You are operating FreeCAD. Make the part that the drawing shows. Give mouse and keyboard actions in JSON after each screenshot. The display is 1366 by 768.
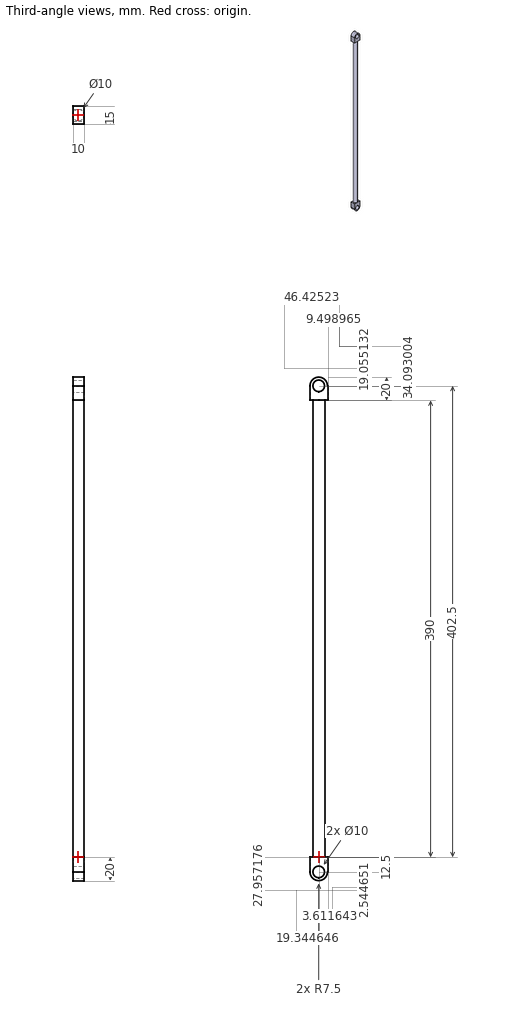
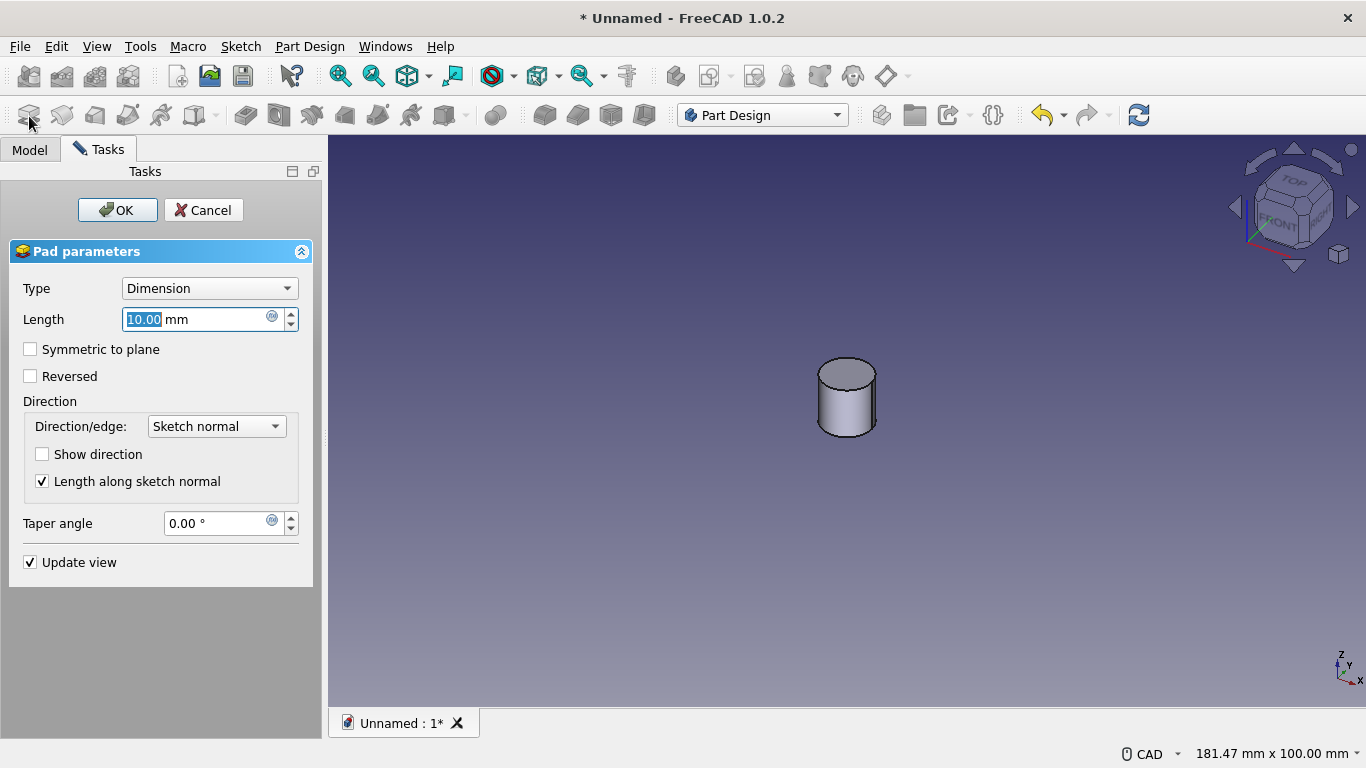
{"action": "type", "text": "390"}
{"action": "key", "text": "Tab"}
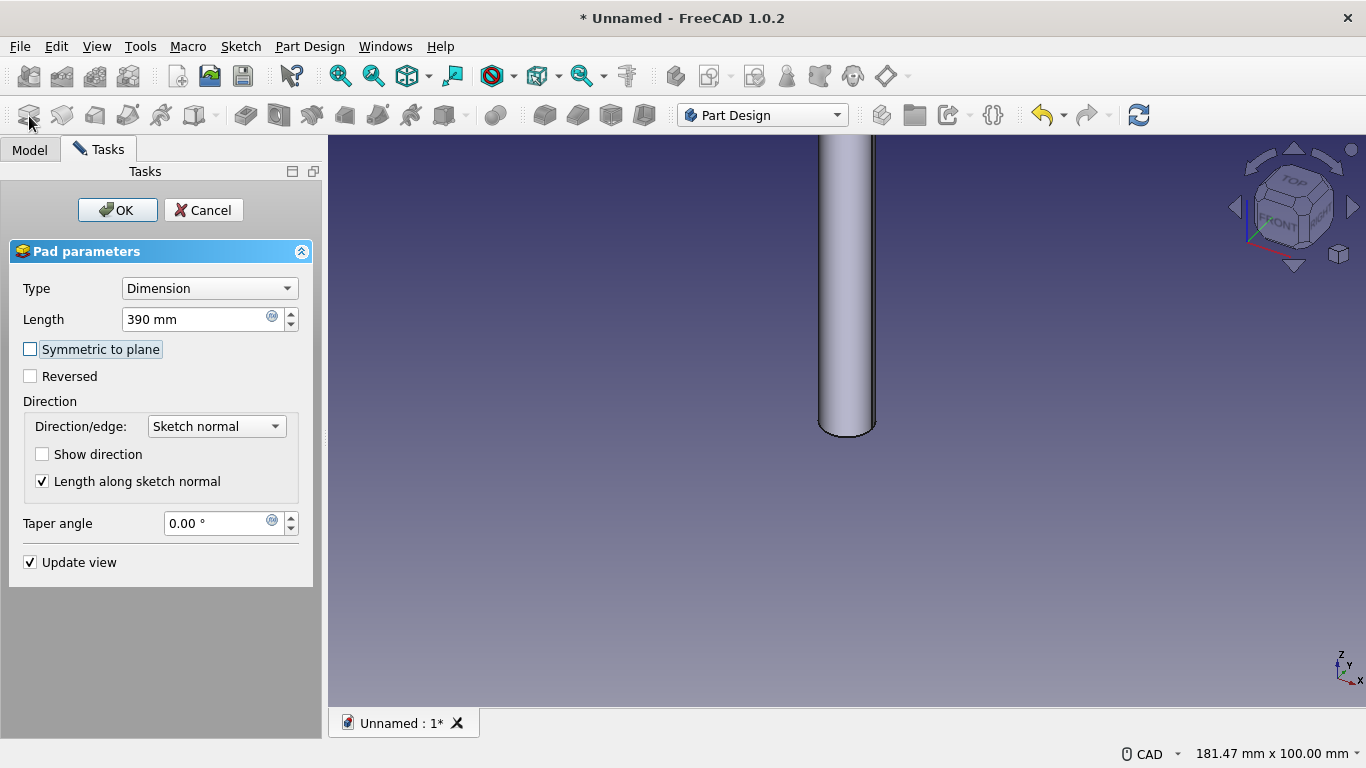
{"action": "left_click", "coordinate": [118, 210]}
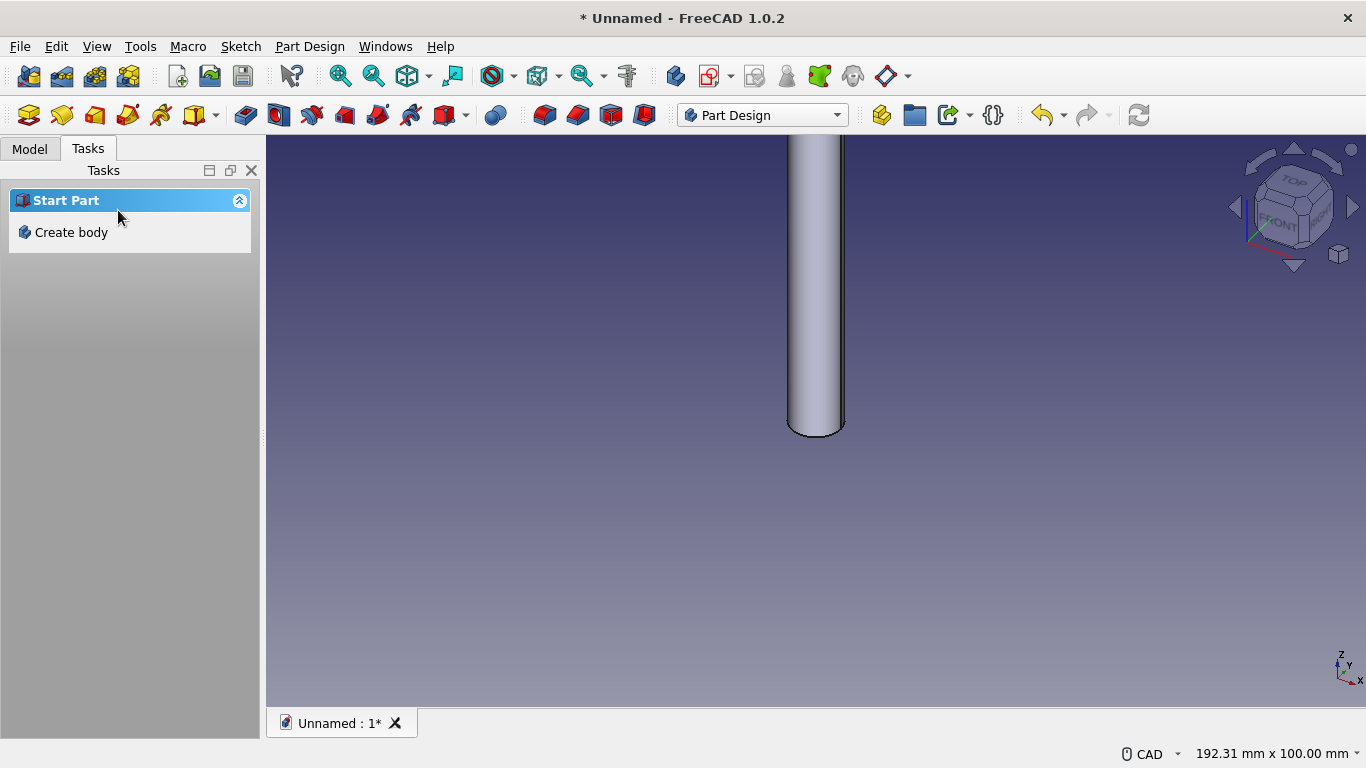
{"action": "left_click", "coordinate": [341, 76]}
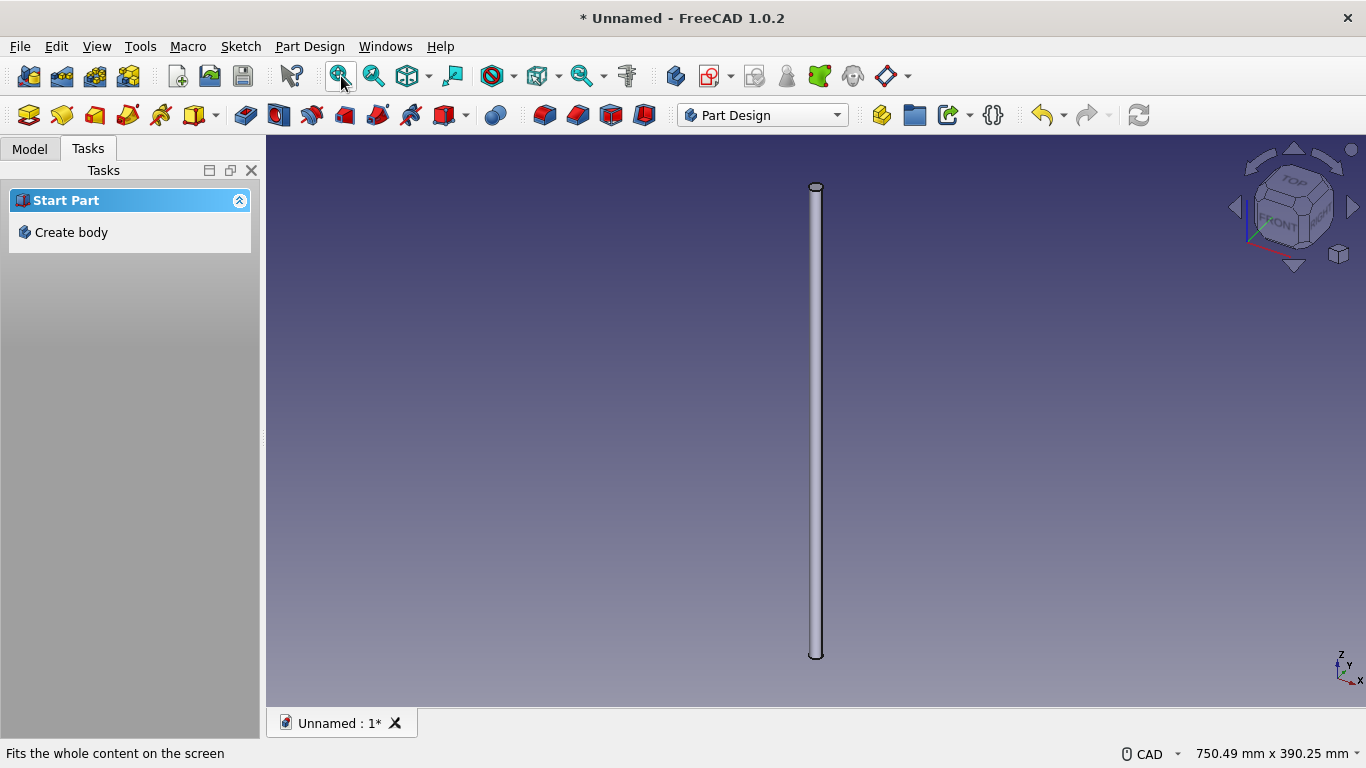
{"action": "key", "text": "5"}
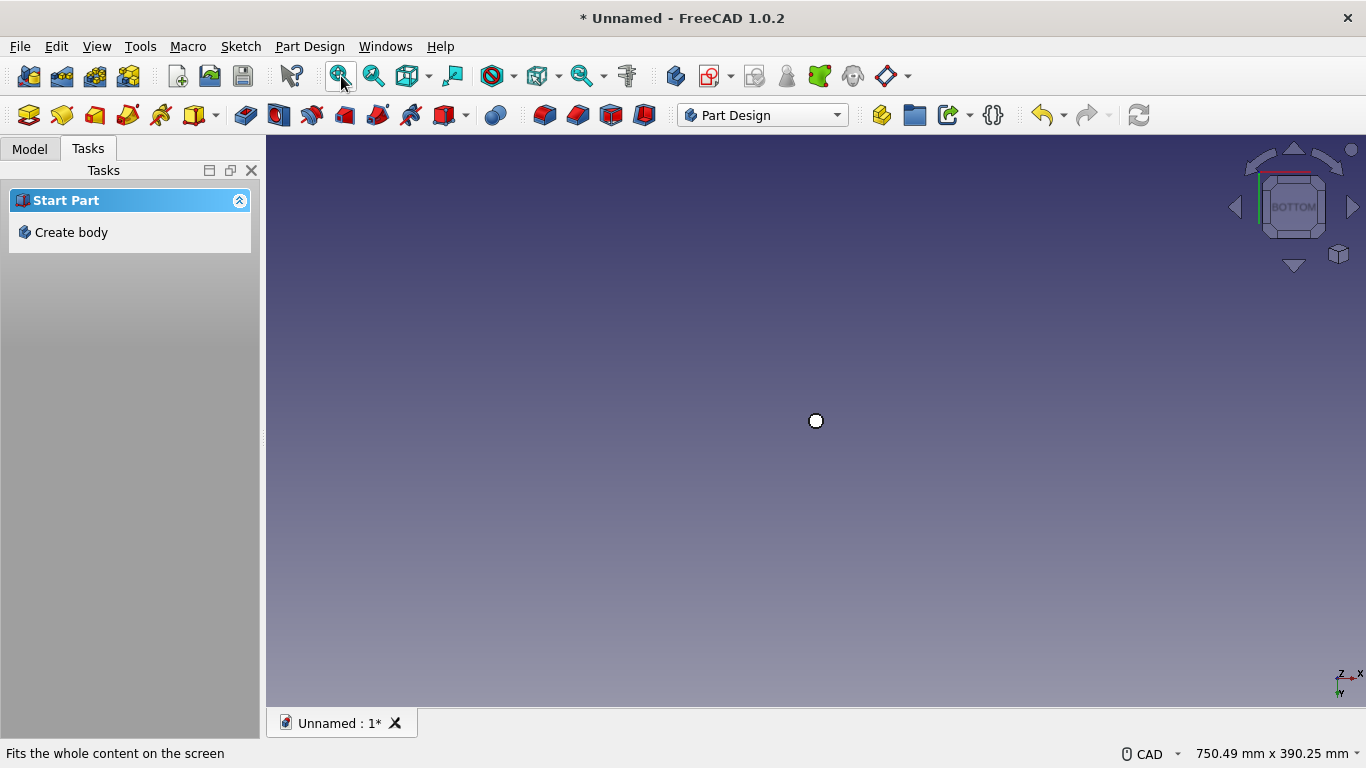
{"action": "left_click", "coordinate": [341, 76]}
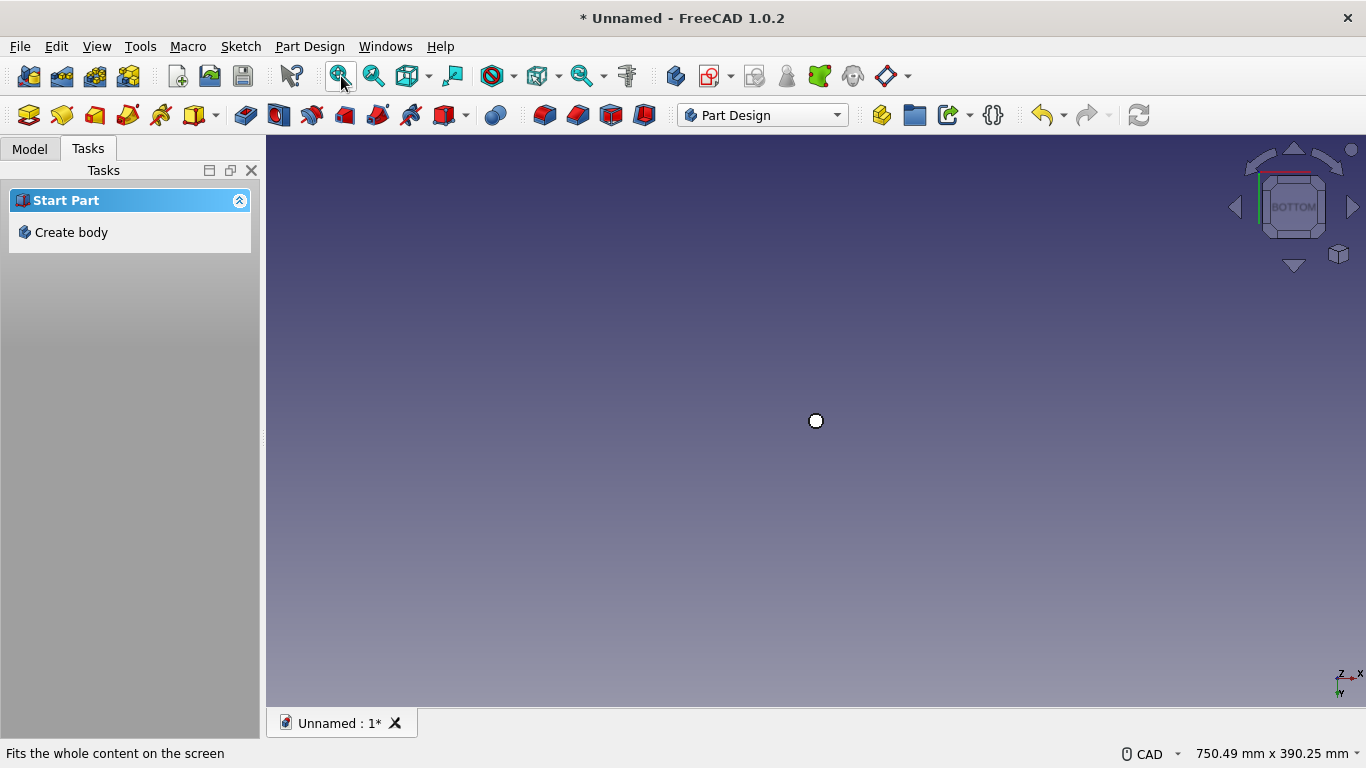
{"action": "key", "text": "1"}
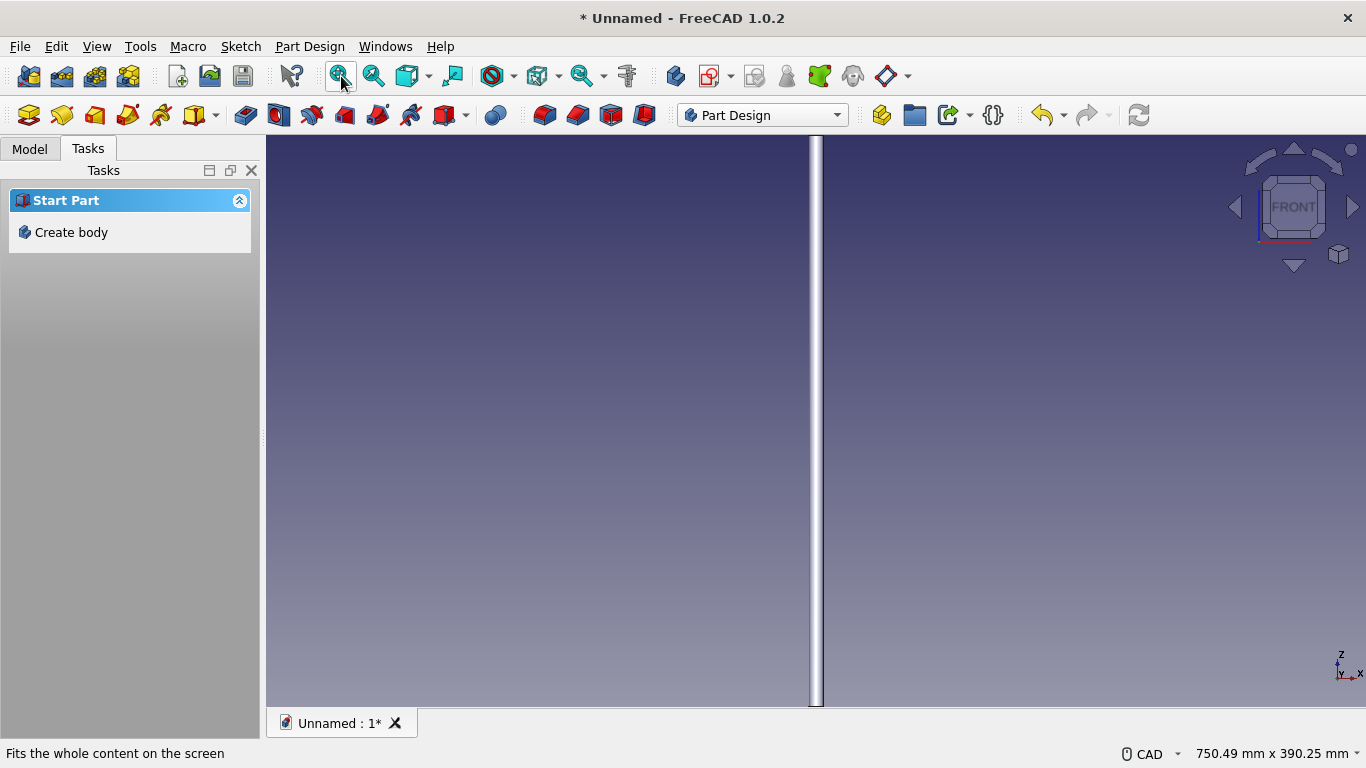
{"action": "left_click", "coordinate": [341, 76]}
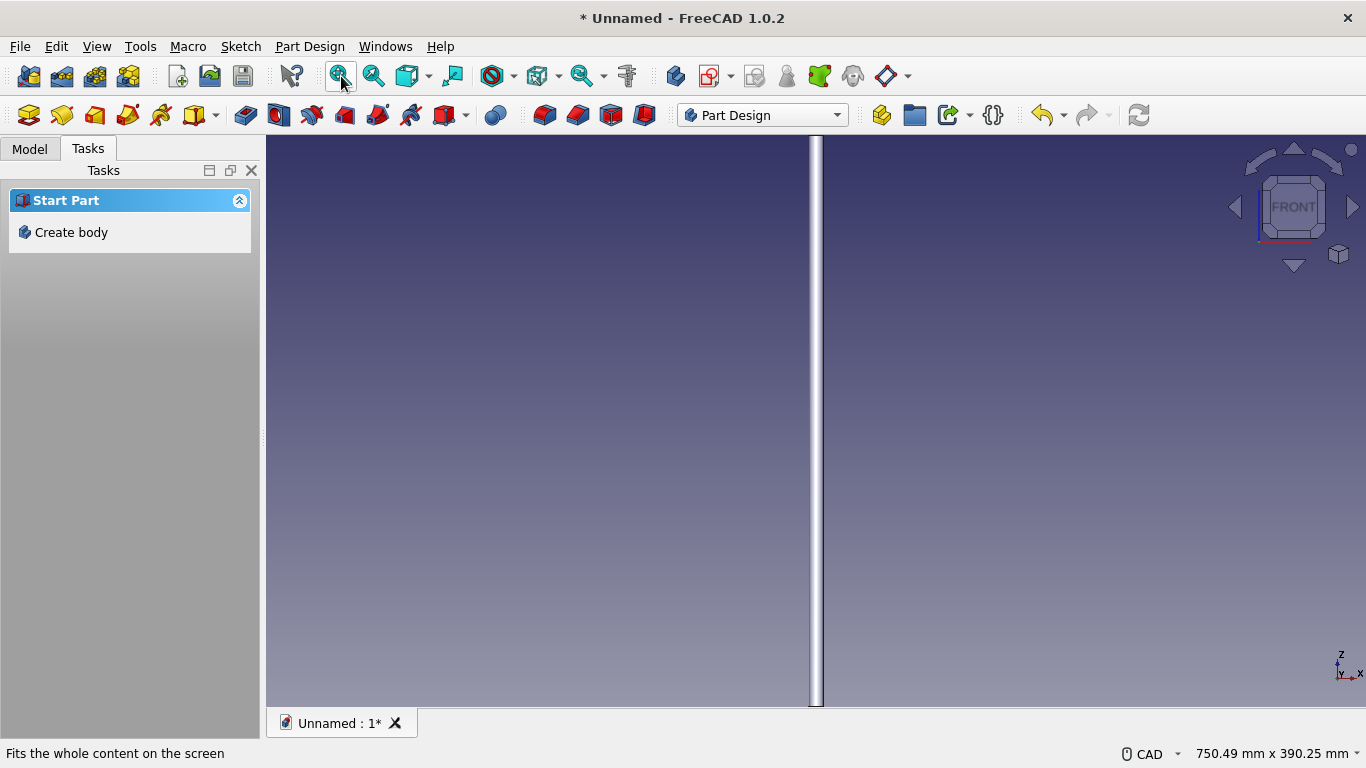
{"action": "key", "text": "3"}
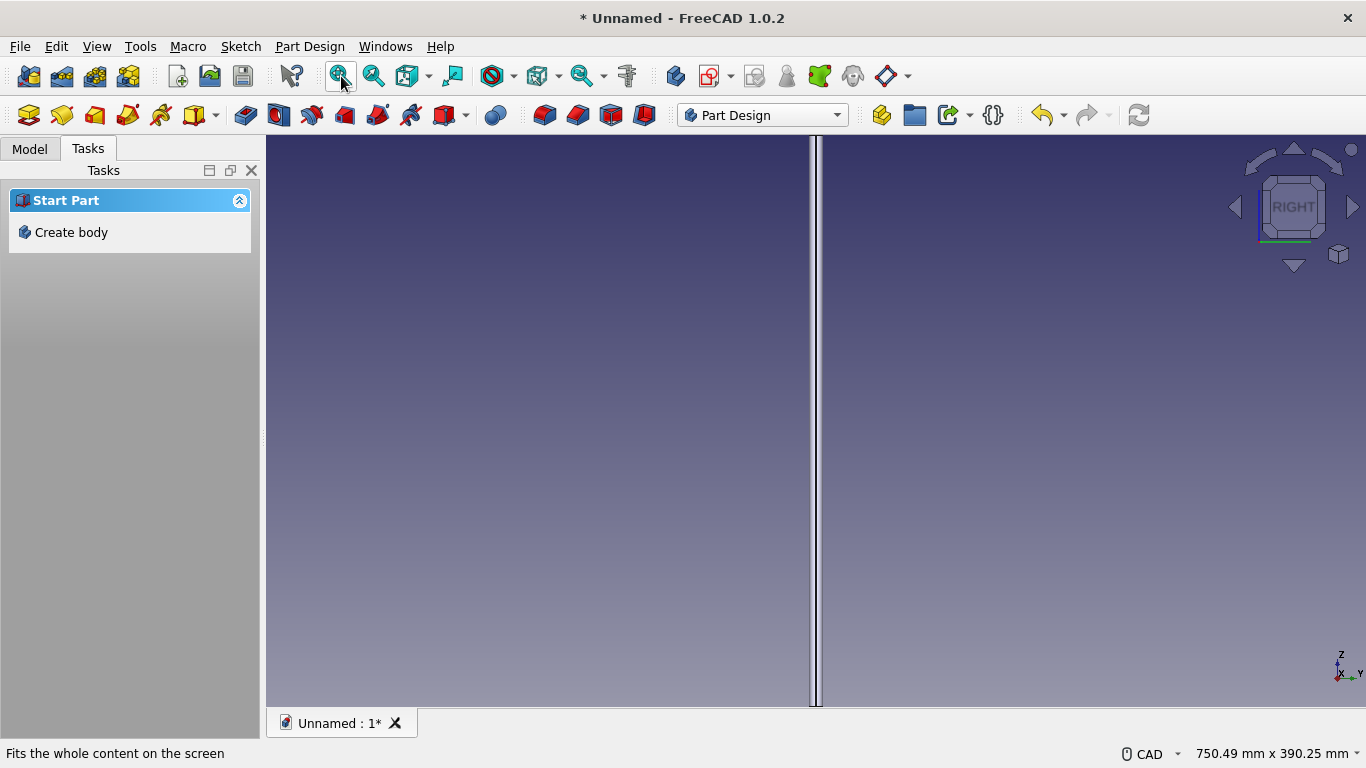
{"action": "left_click", "coordinate": [341, 76]}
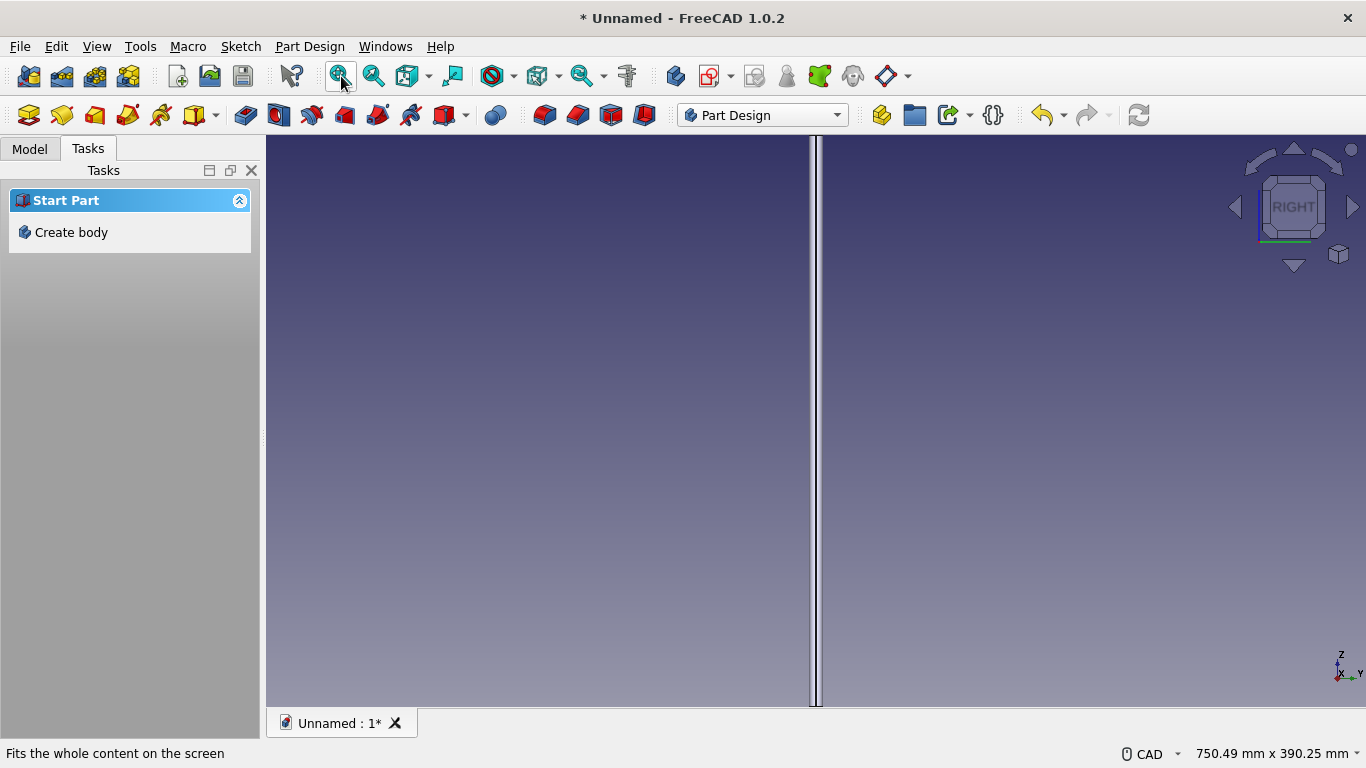
{"action": "left_click", "coordinate": [708, 76]}